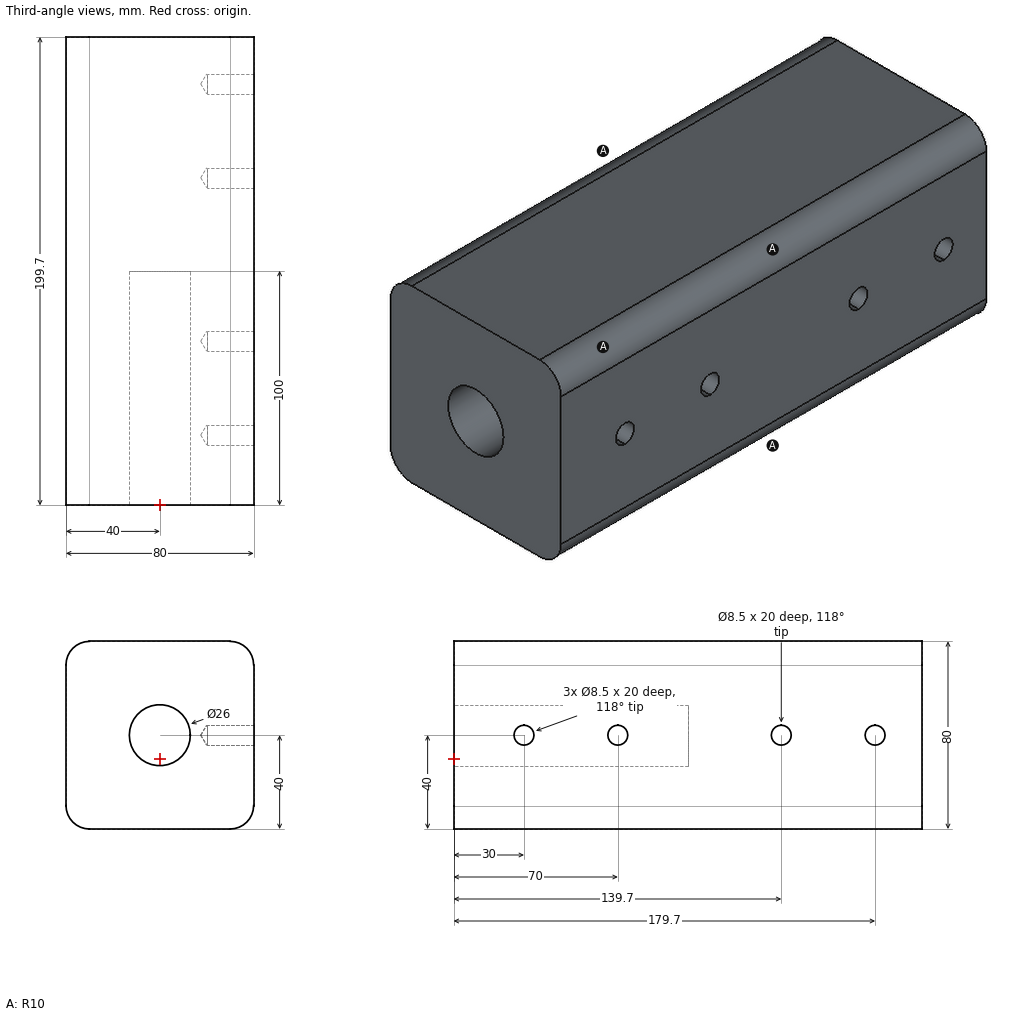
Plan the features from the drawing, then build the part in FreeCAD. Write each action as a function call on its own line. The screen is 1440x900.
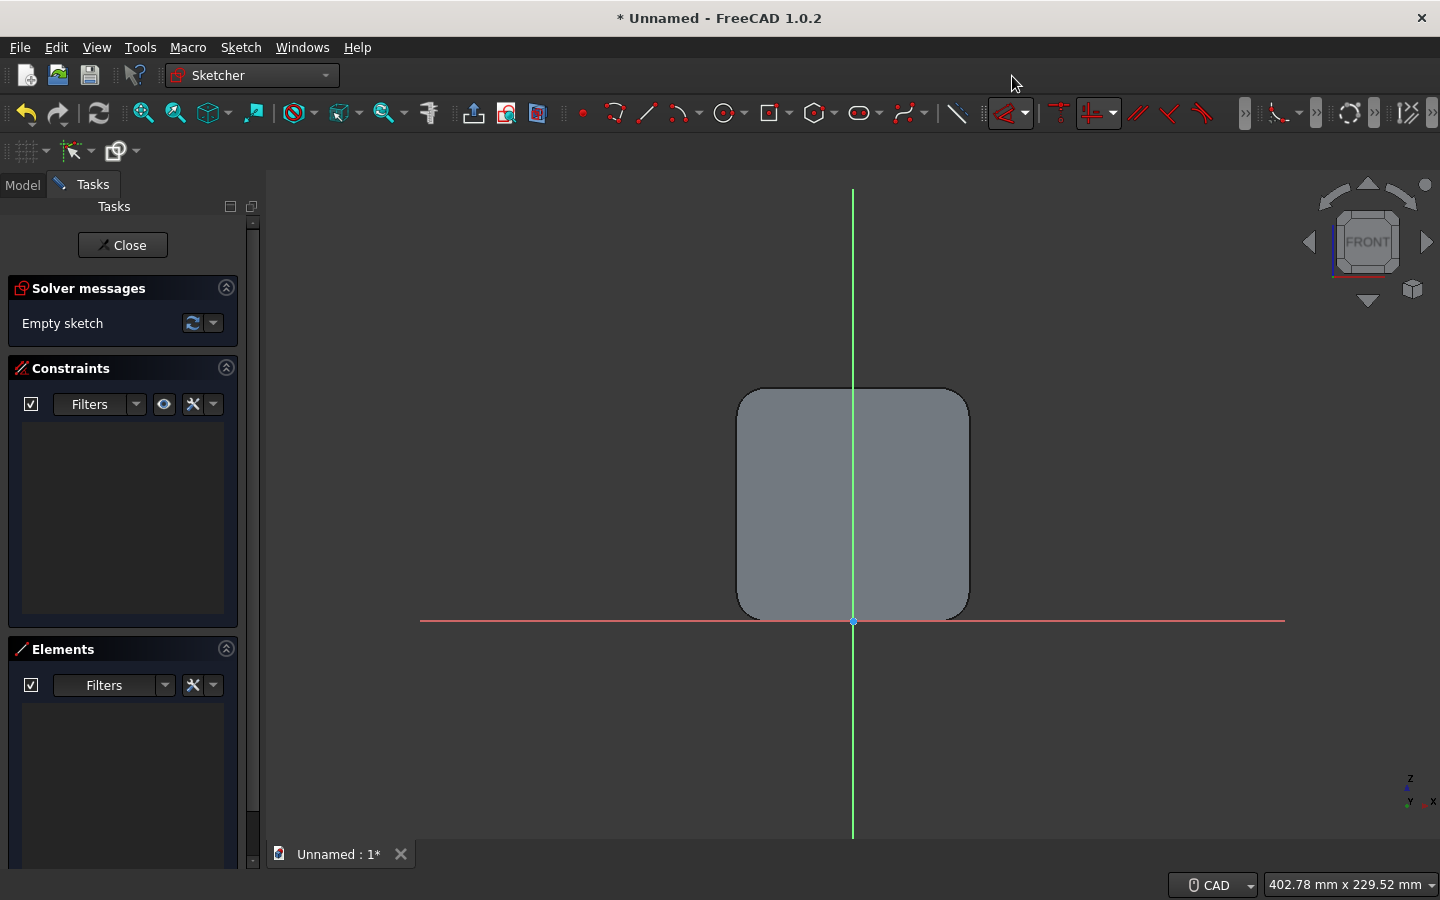
scroll(893, 567, up, 5)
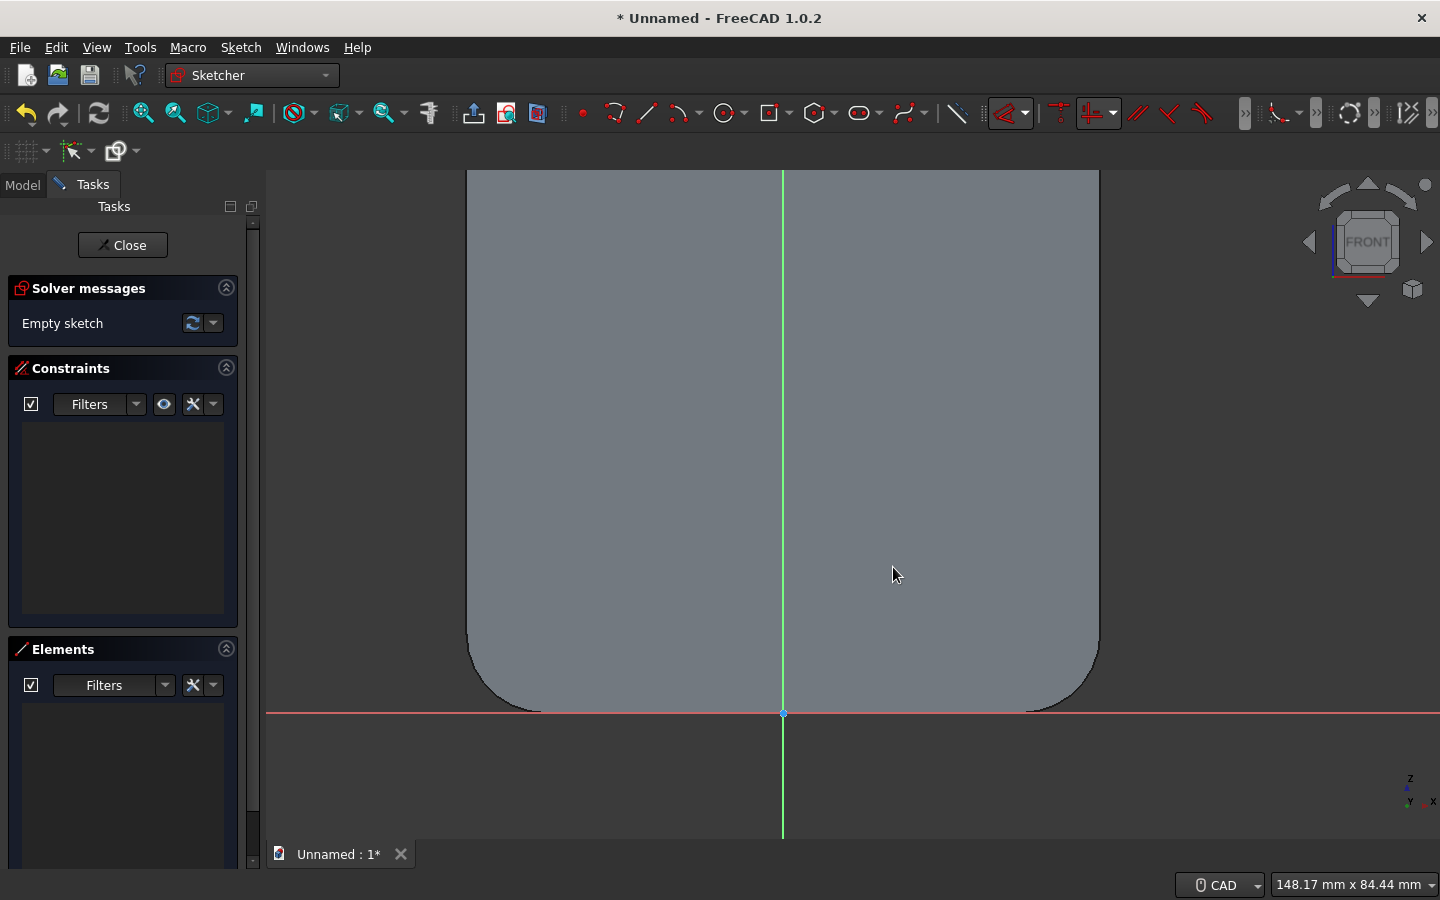
click(724, 114)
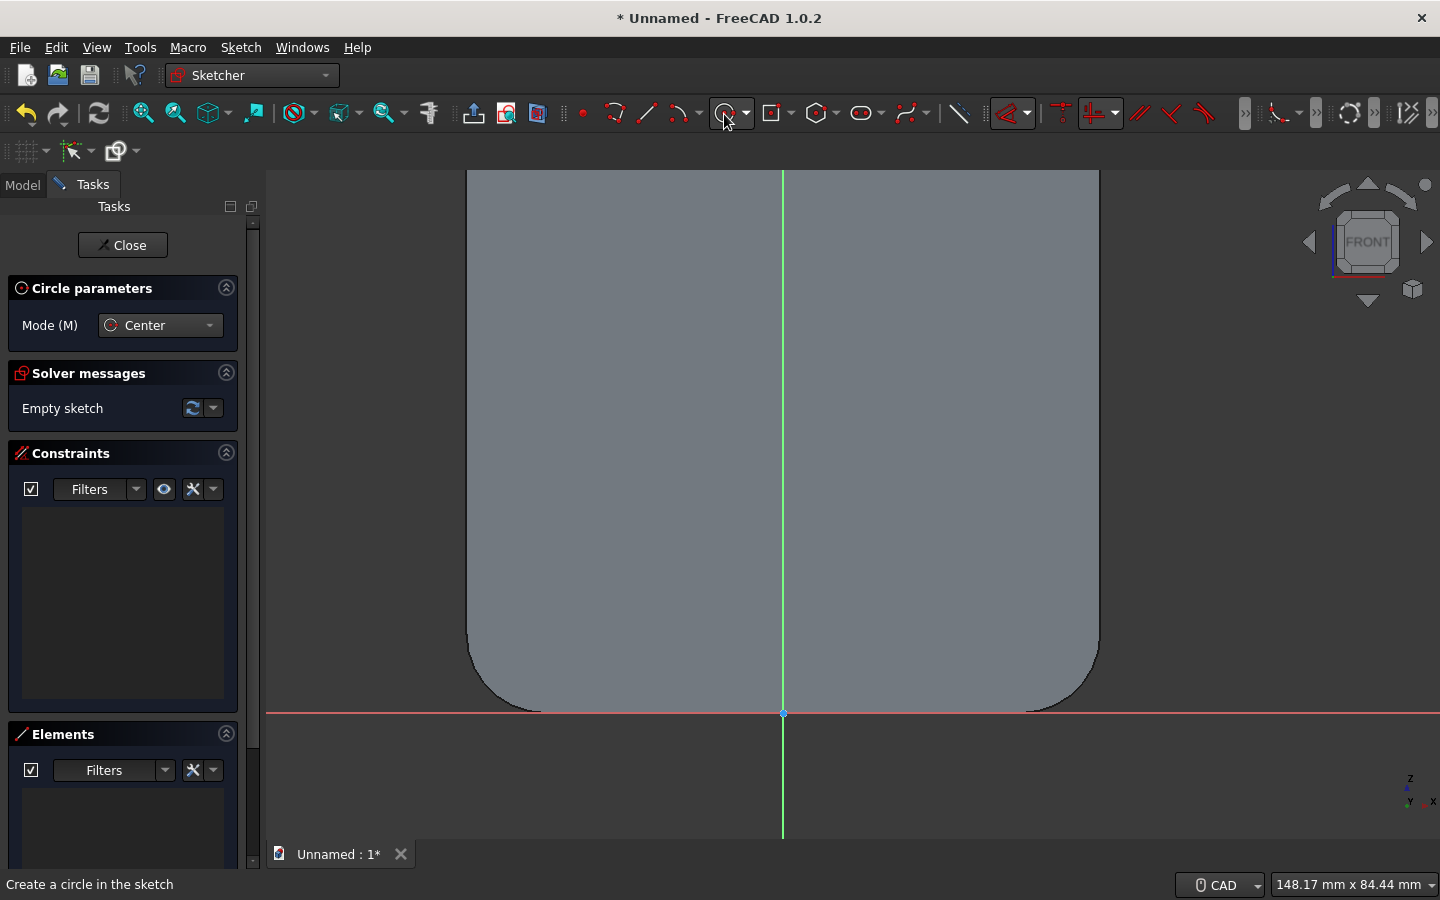
click(783, 396)
click(856, 323)
key(Escape)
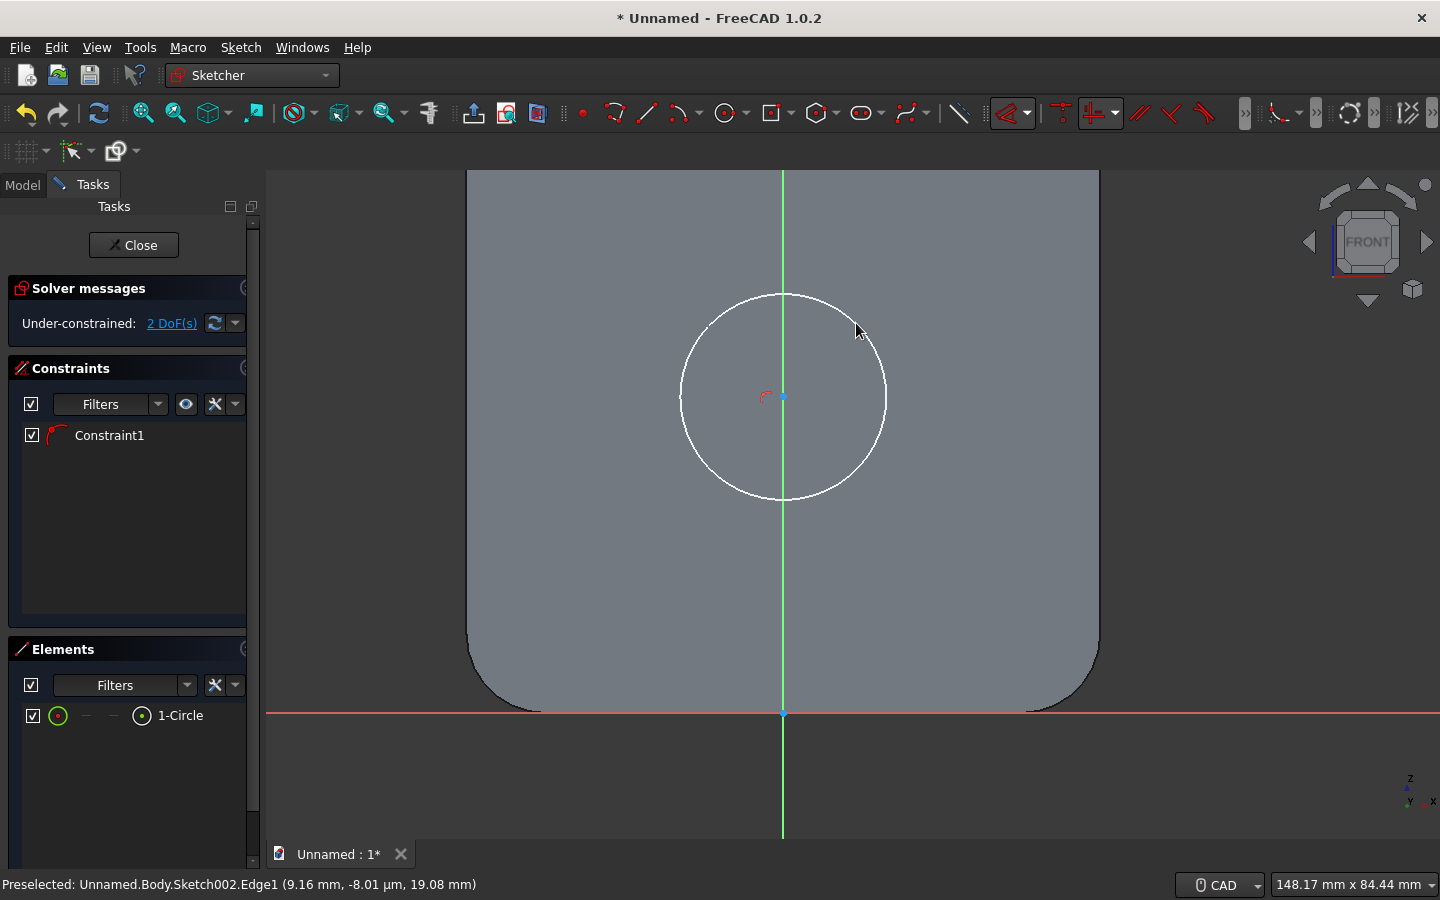
click(856, 324)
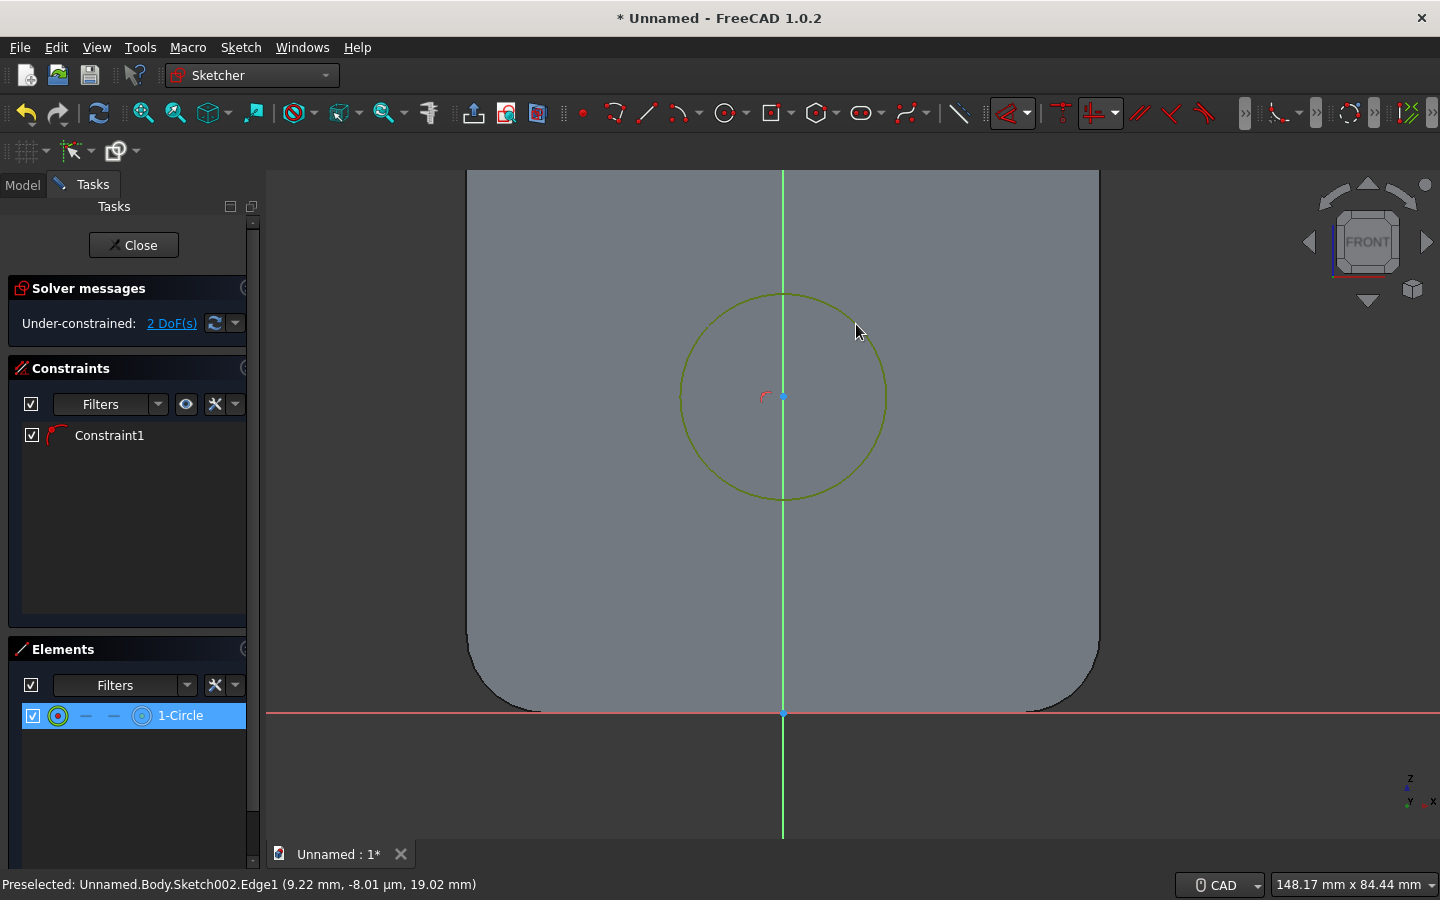
click(1030, 114)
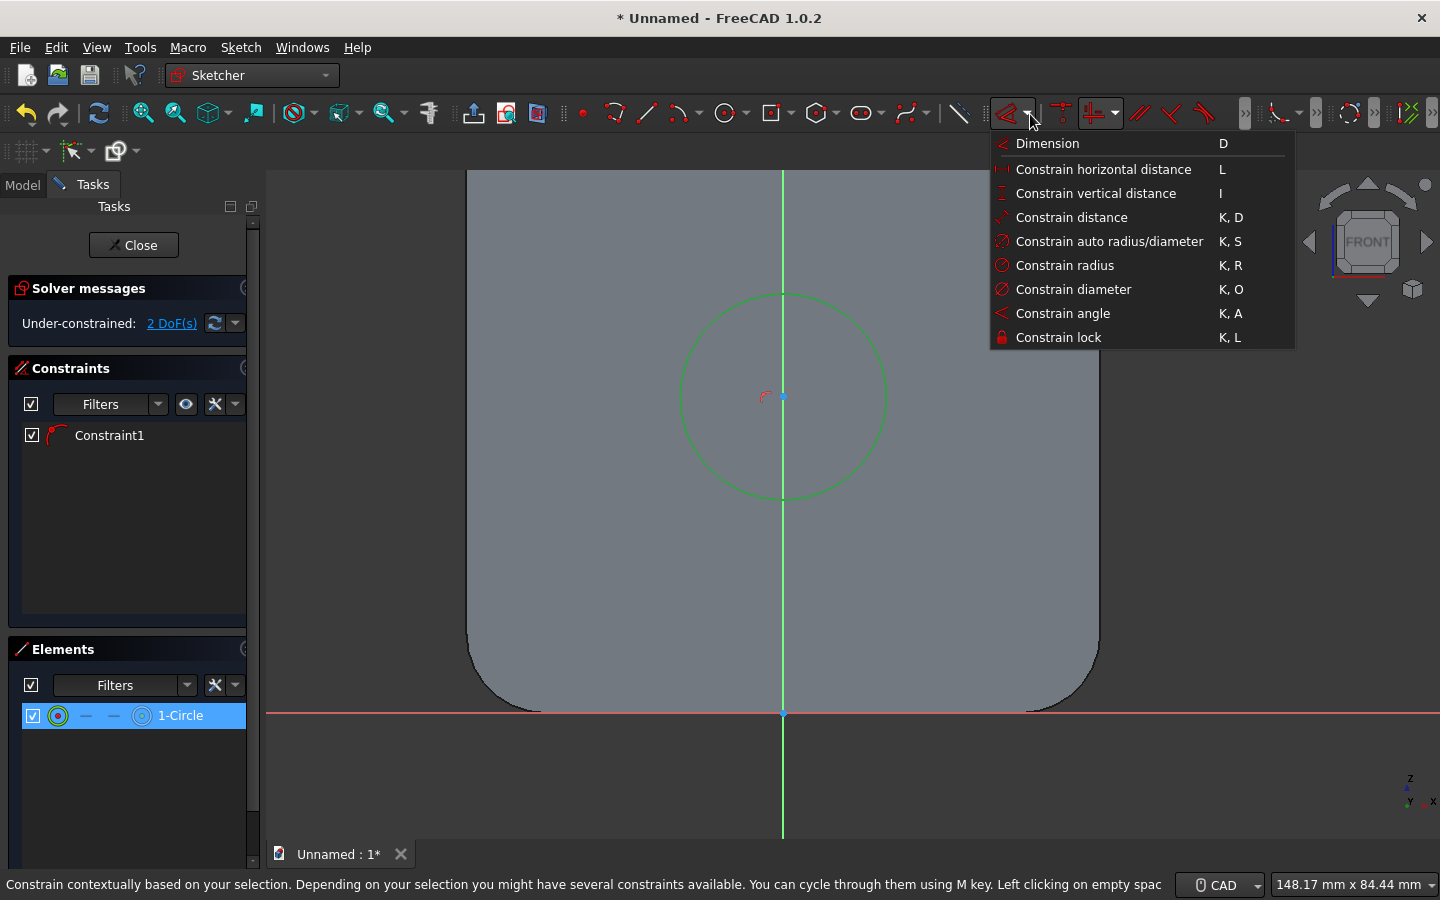
click(1143, 289)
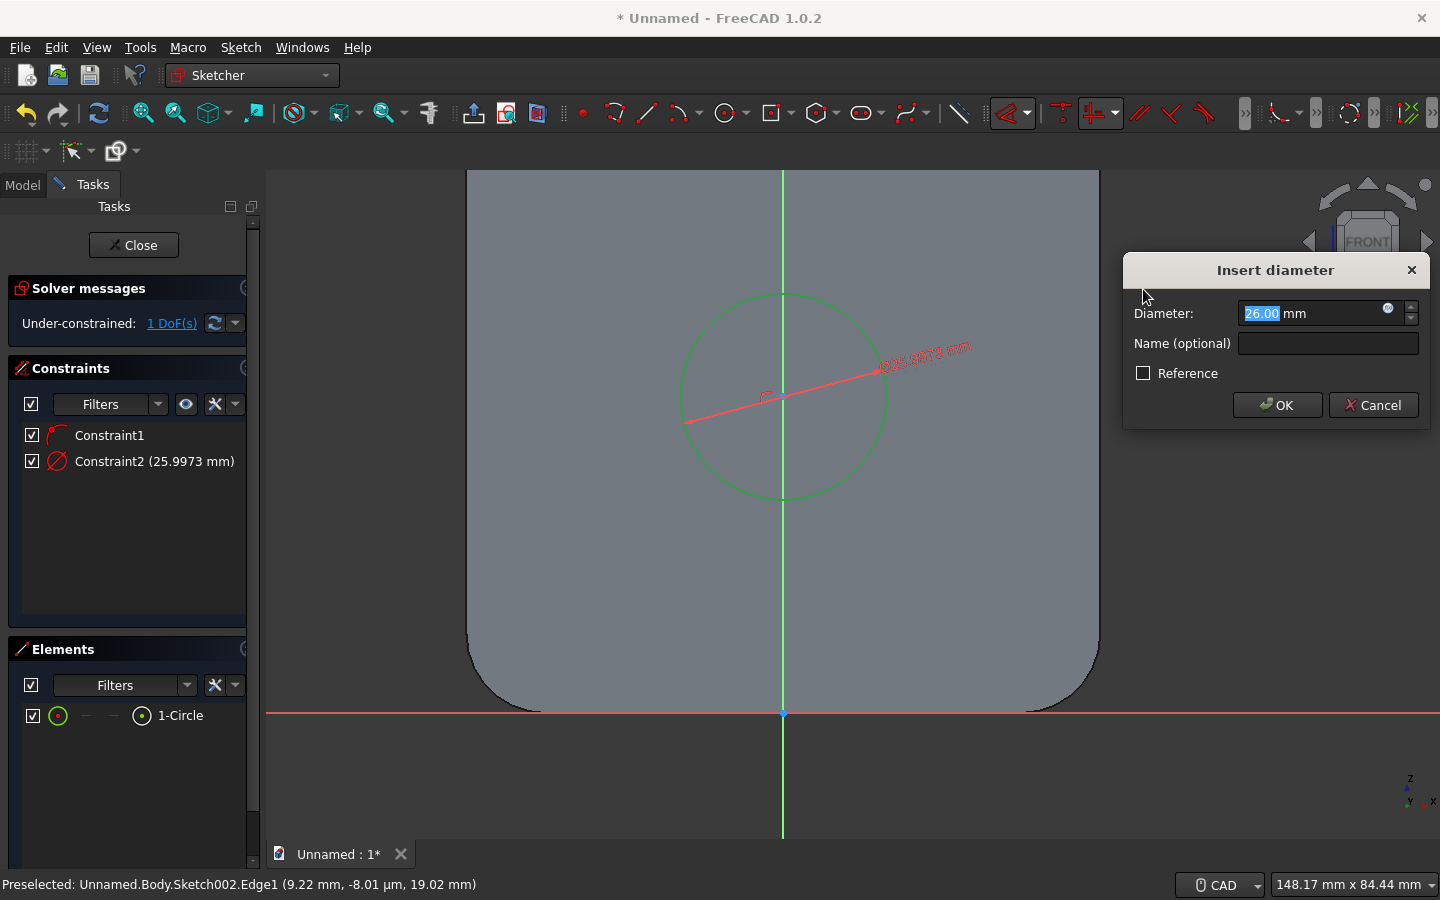
text(26)
key(Return)